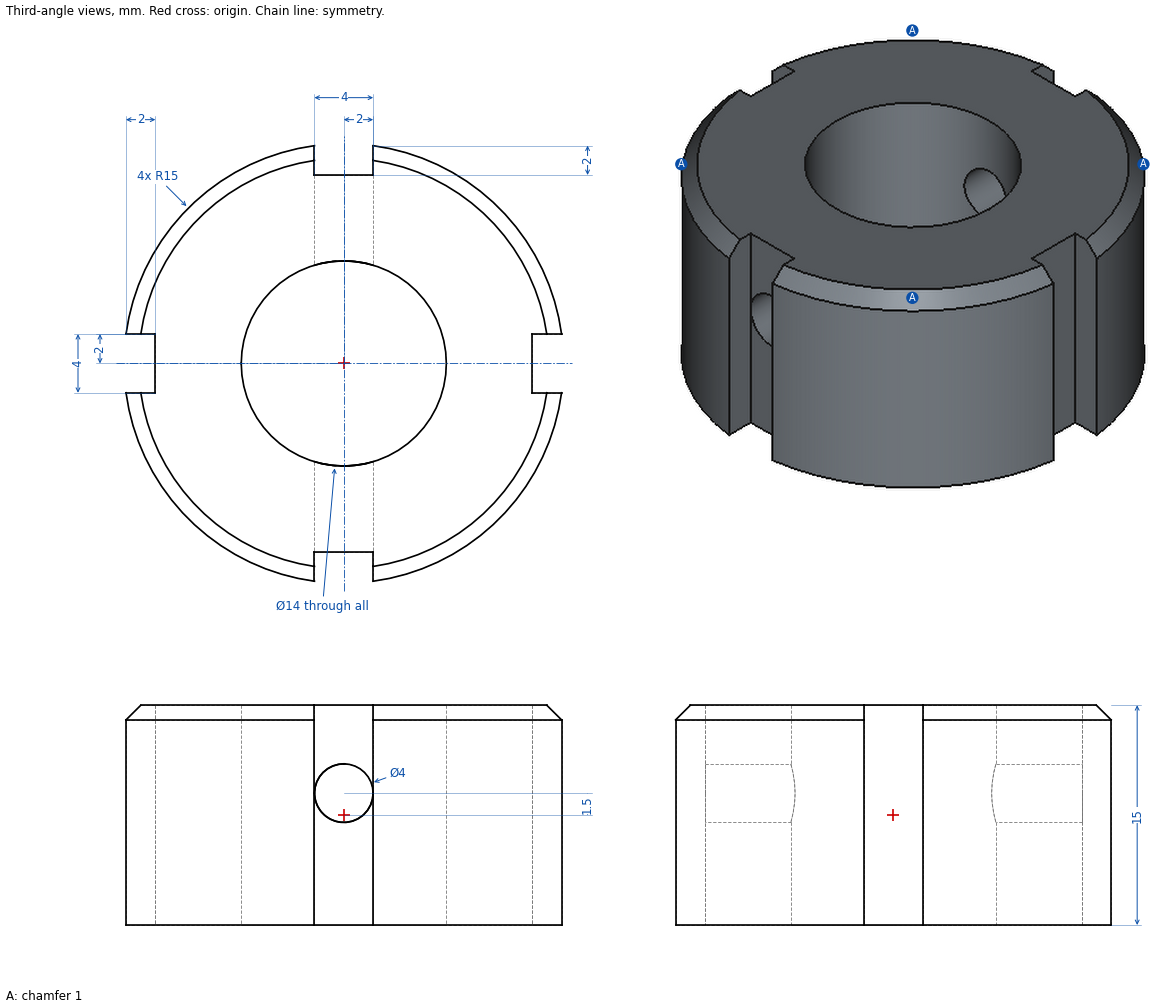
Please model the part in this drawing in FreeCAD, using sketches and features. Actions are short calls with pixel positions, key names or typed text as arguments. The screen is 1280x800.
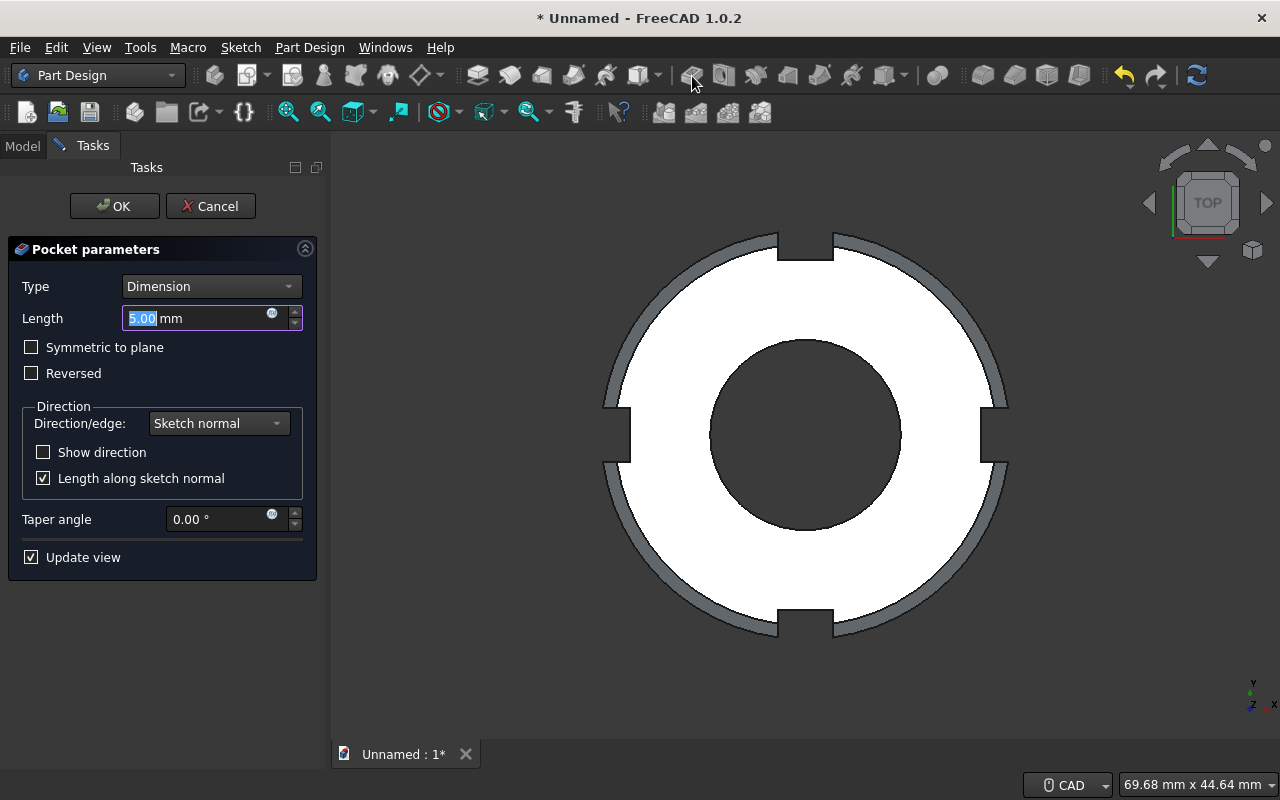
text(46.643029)
key(Tab)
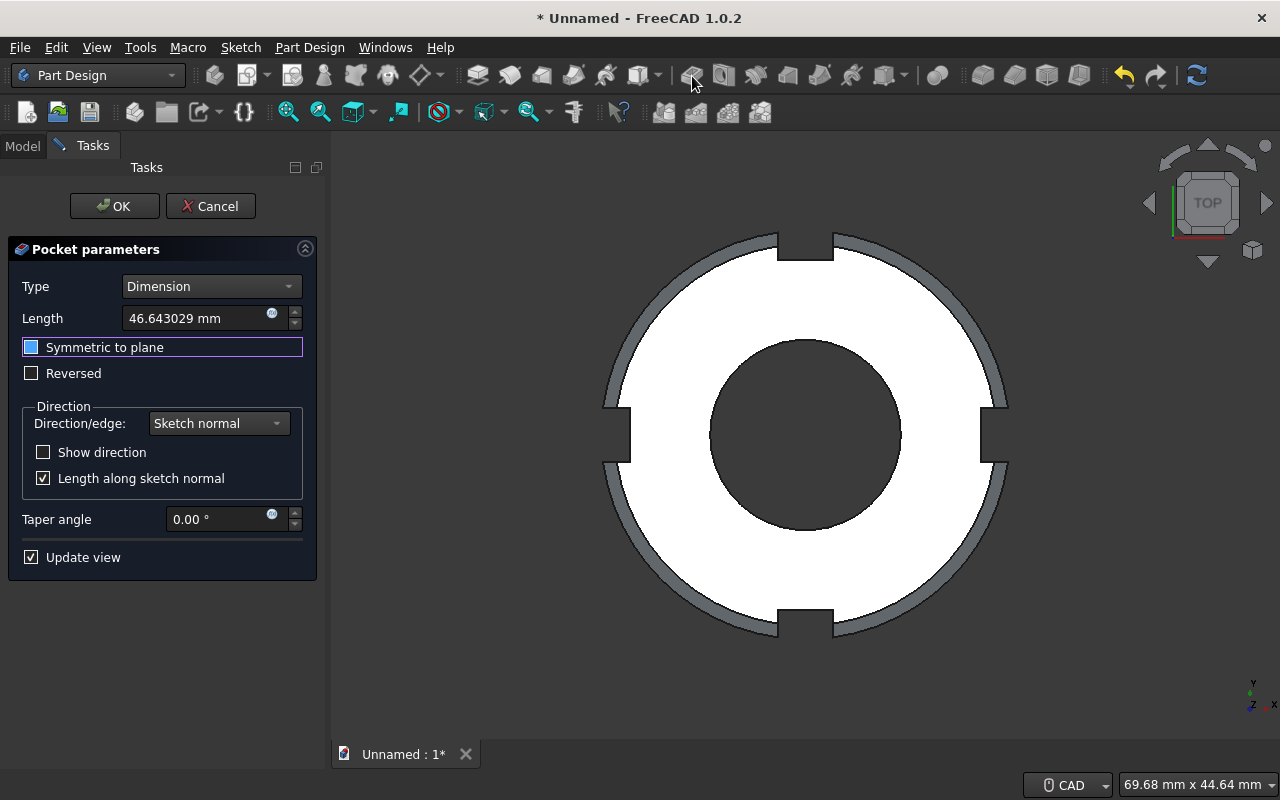
click(30, 347)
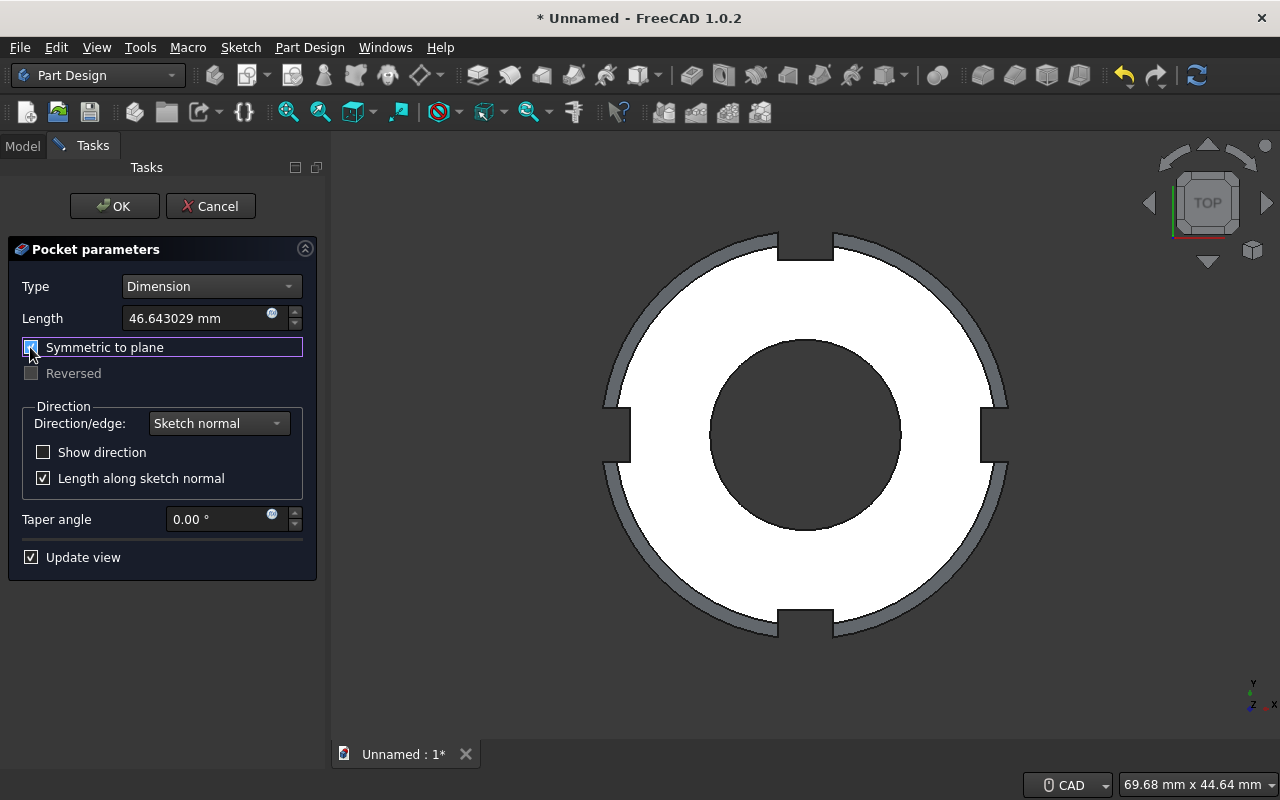
click(115, 206)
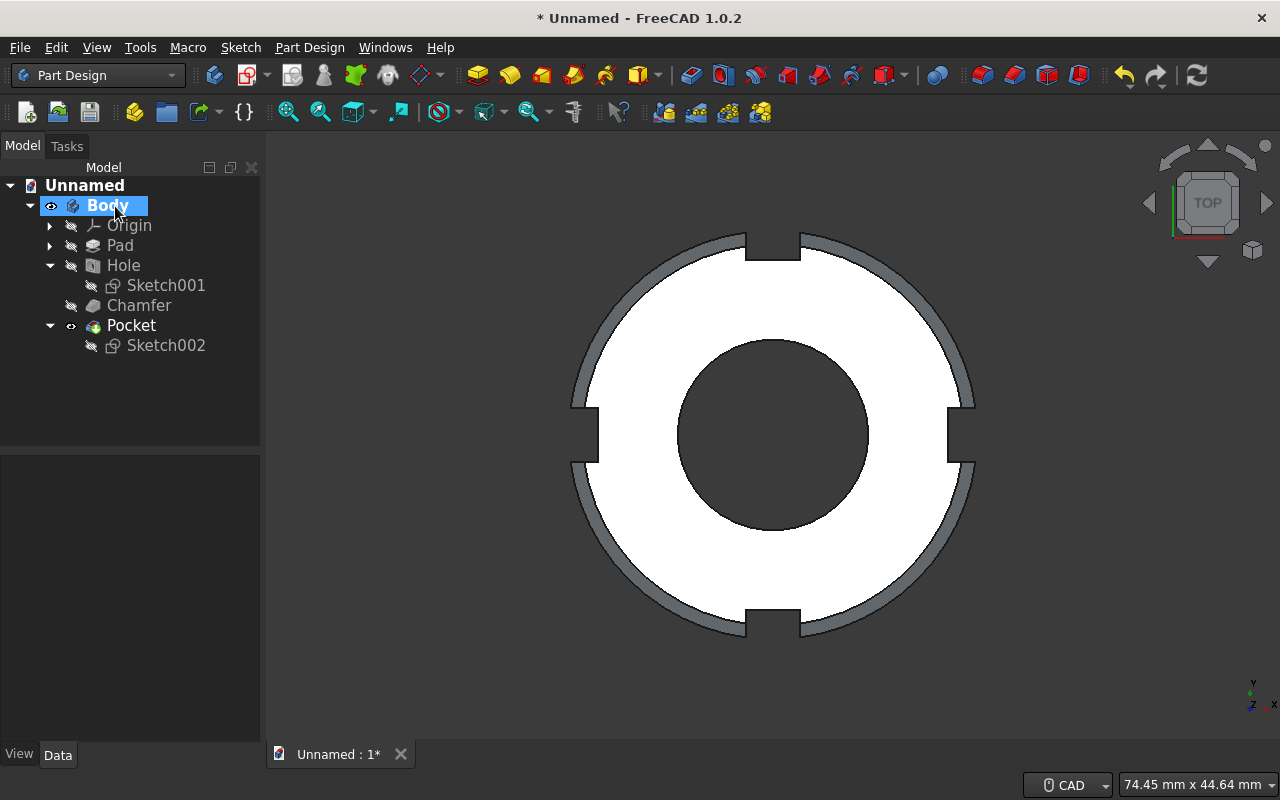
key(0)